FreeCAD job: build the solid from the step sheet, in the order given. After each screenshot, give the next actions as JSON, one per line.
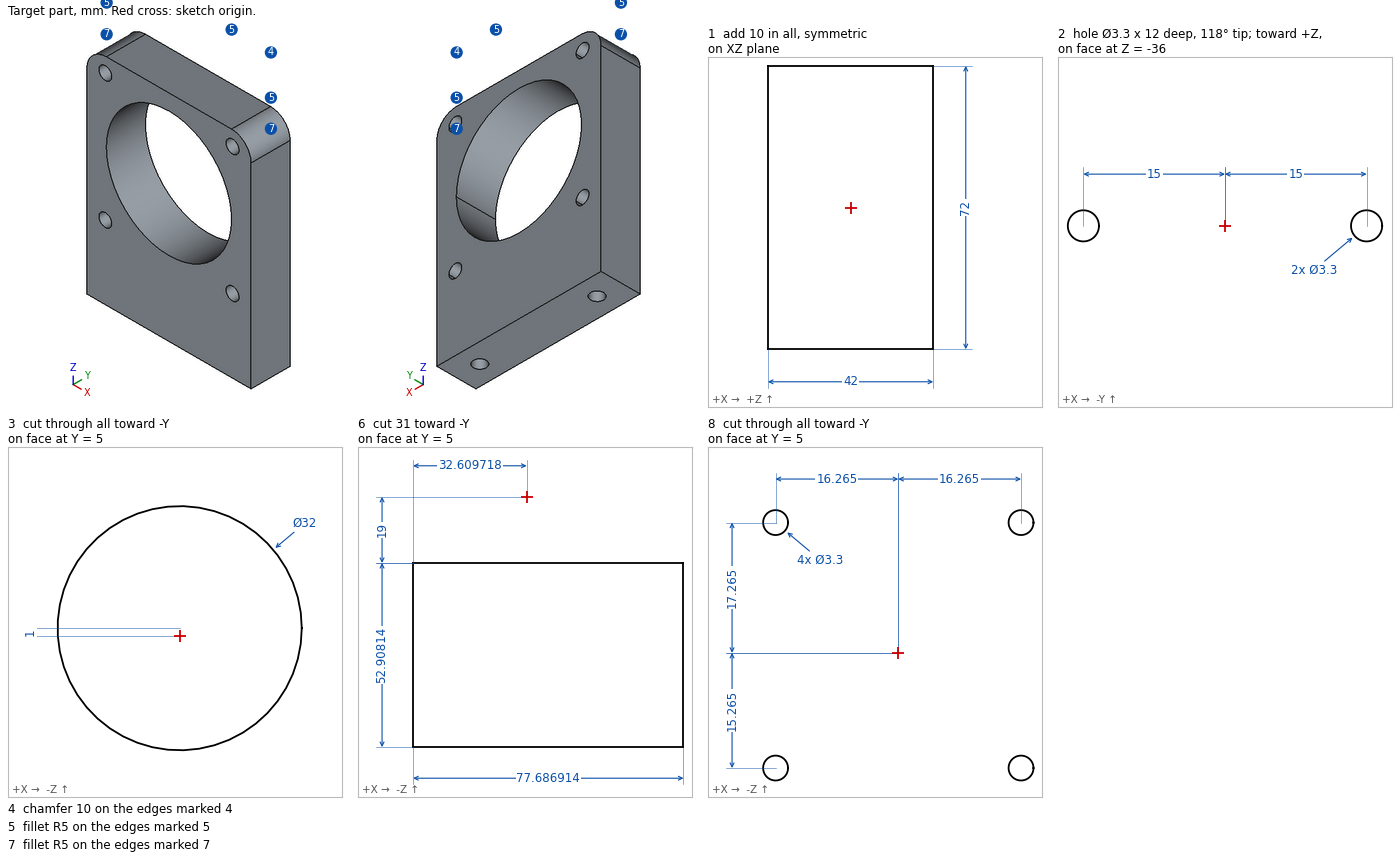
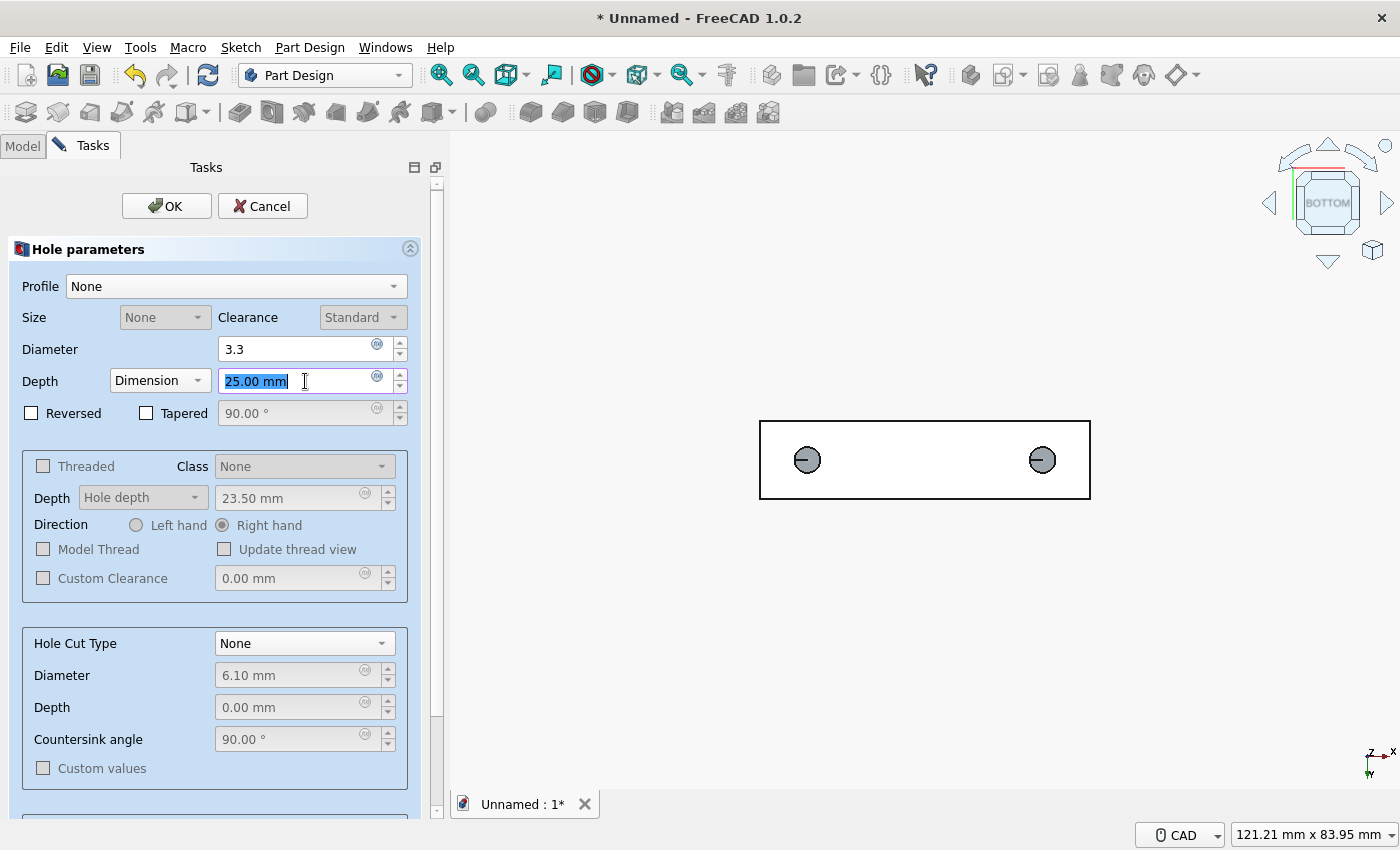
{"action": "type", "text": "12"}
{"action": "key", "text": "Tab"}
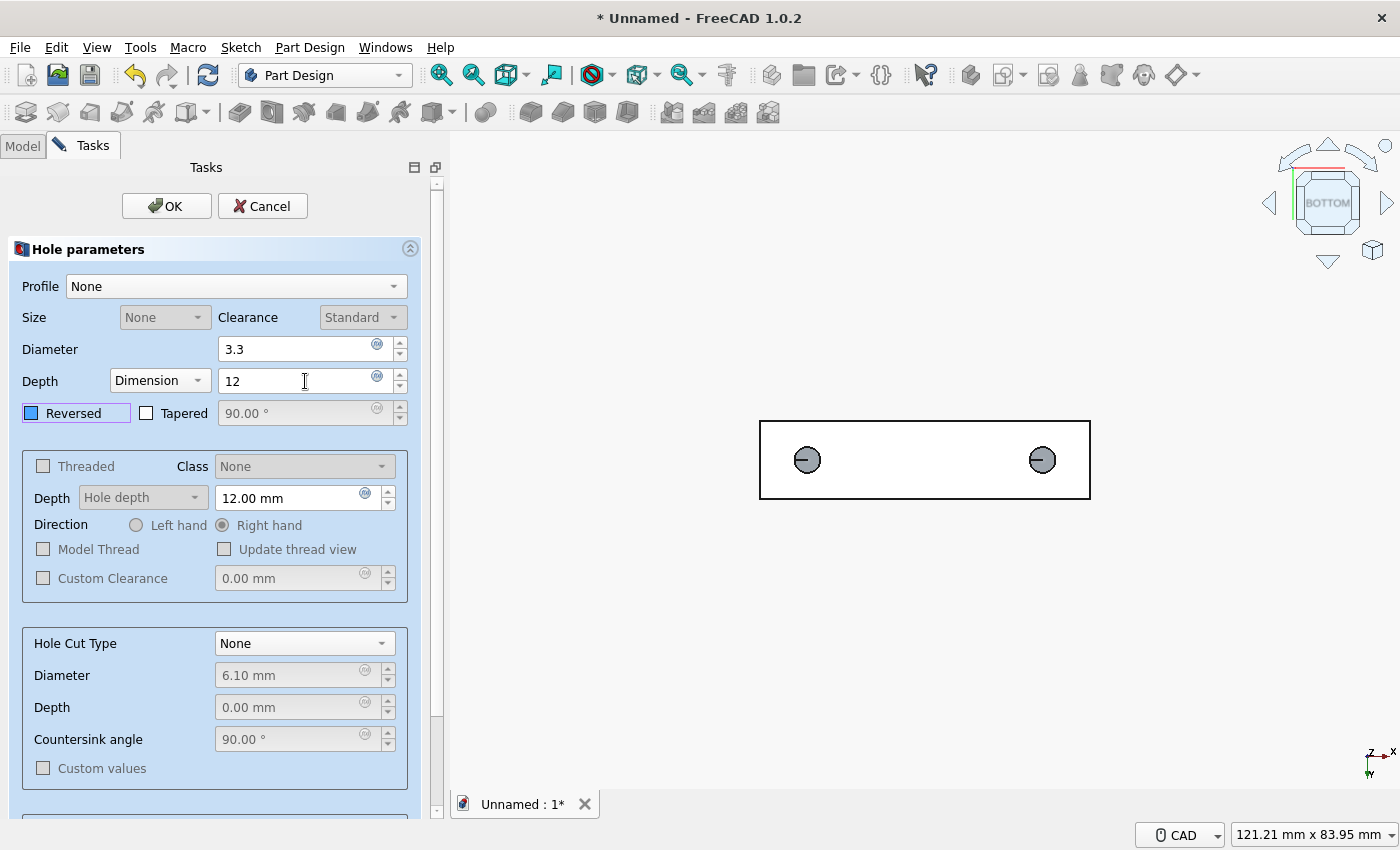
{"action": "left_click", "coordinate": [167, 206]}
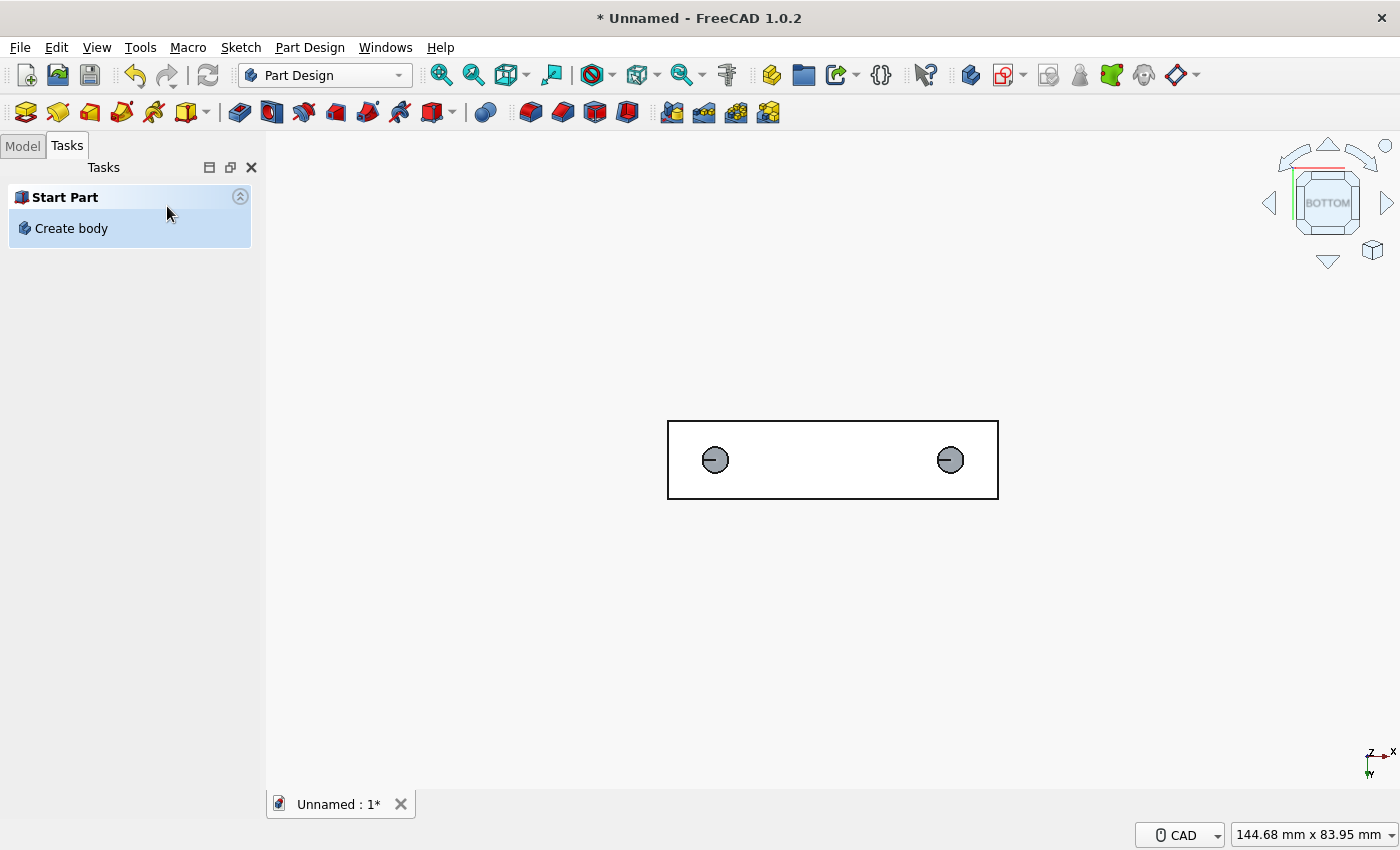
{"action": "left_click", "coordinate": [442, 76]}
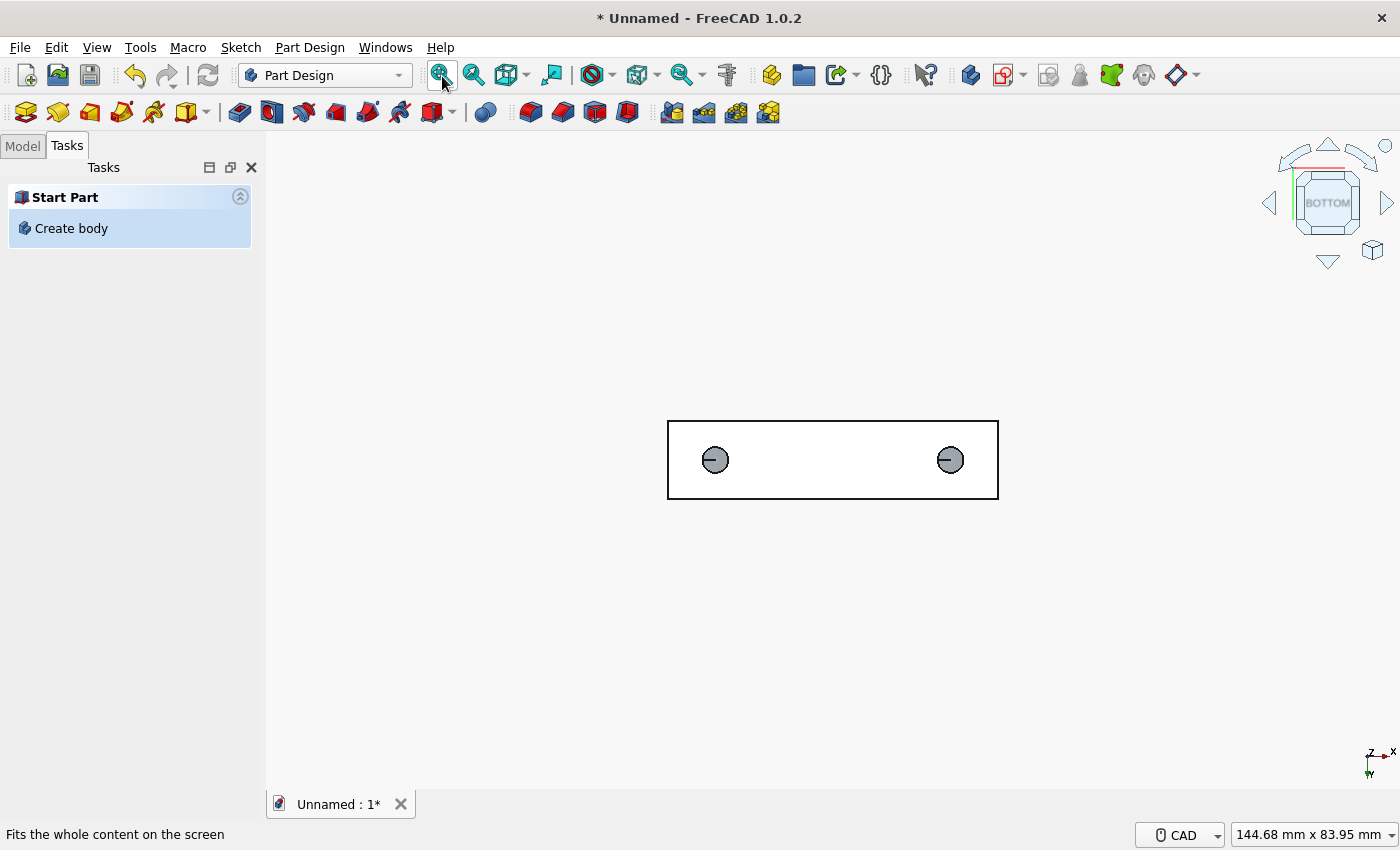
{"action": "key", "text": "4"}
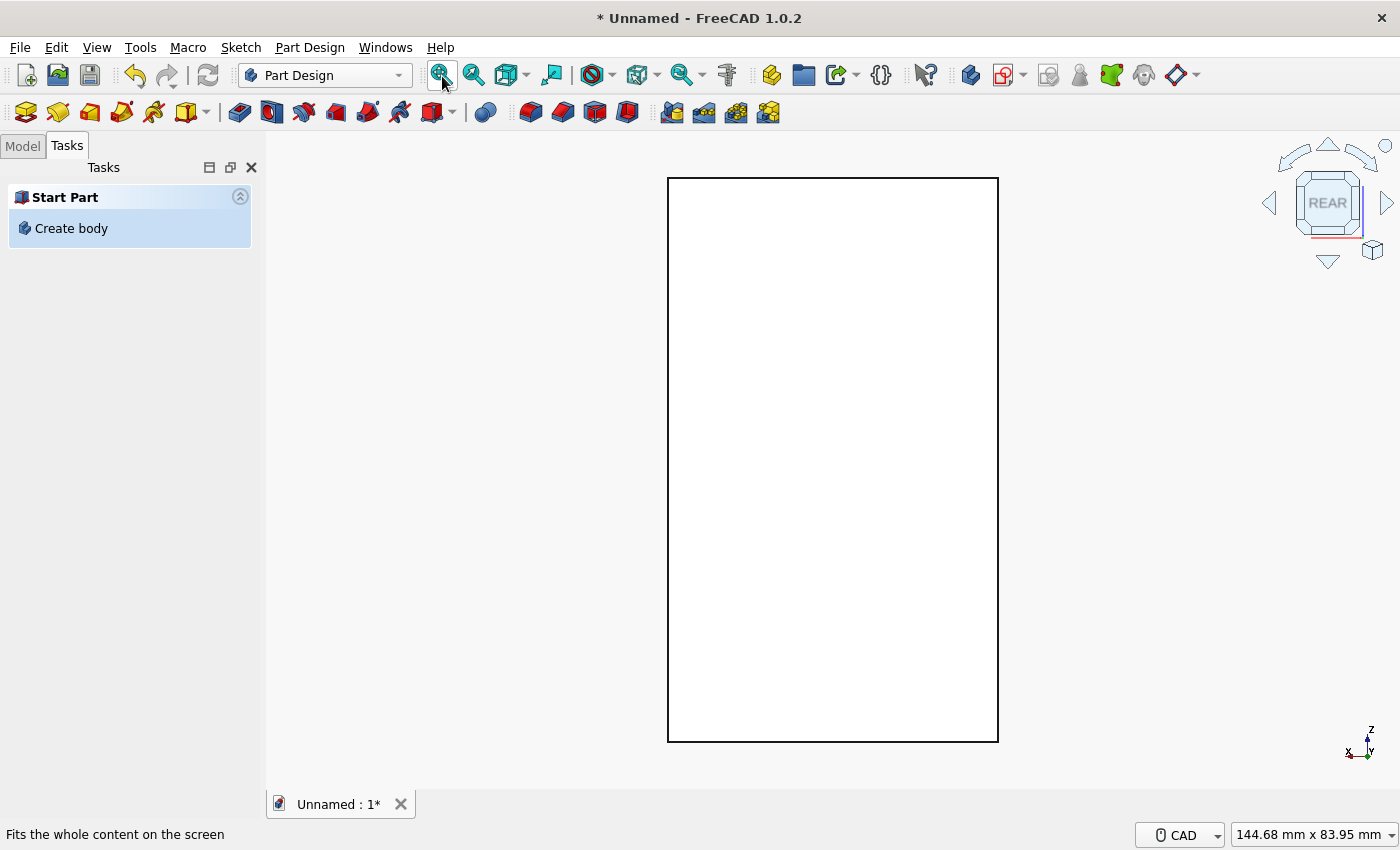
{"action": "left_click", "coordinate": [833, 378]}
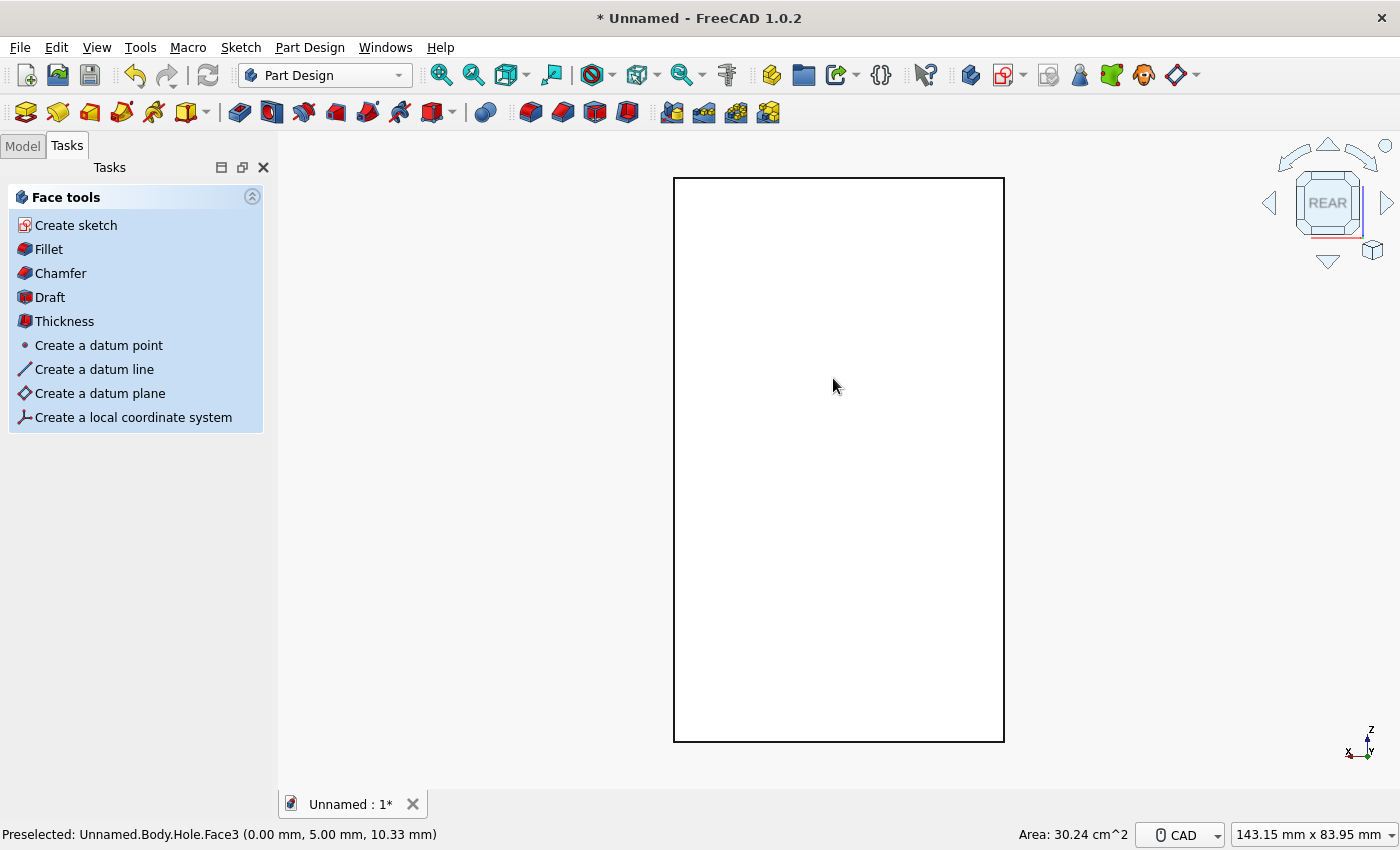
{"action": "left_click", "coordinate": [1004, 76]}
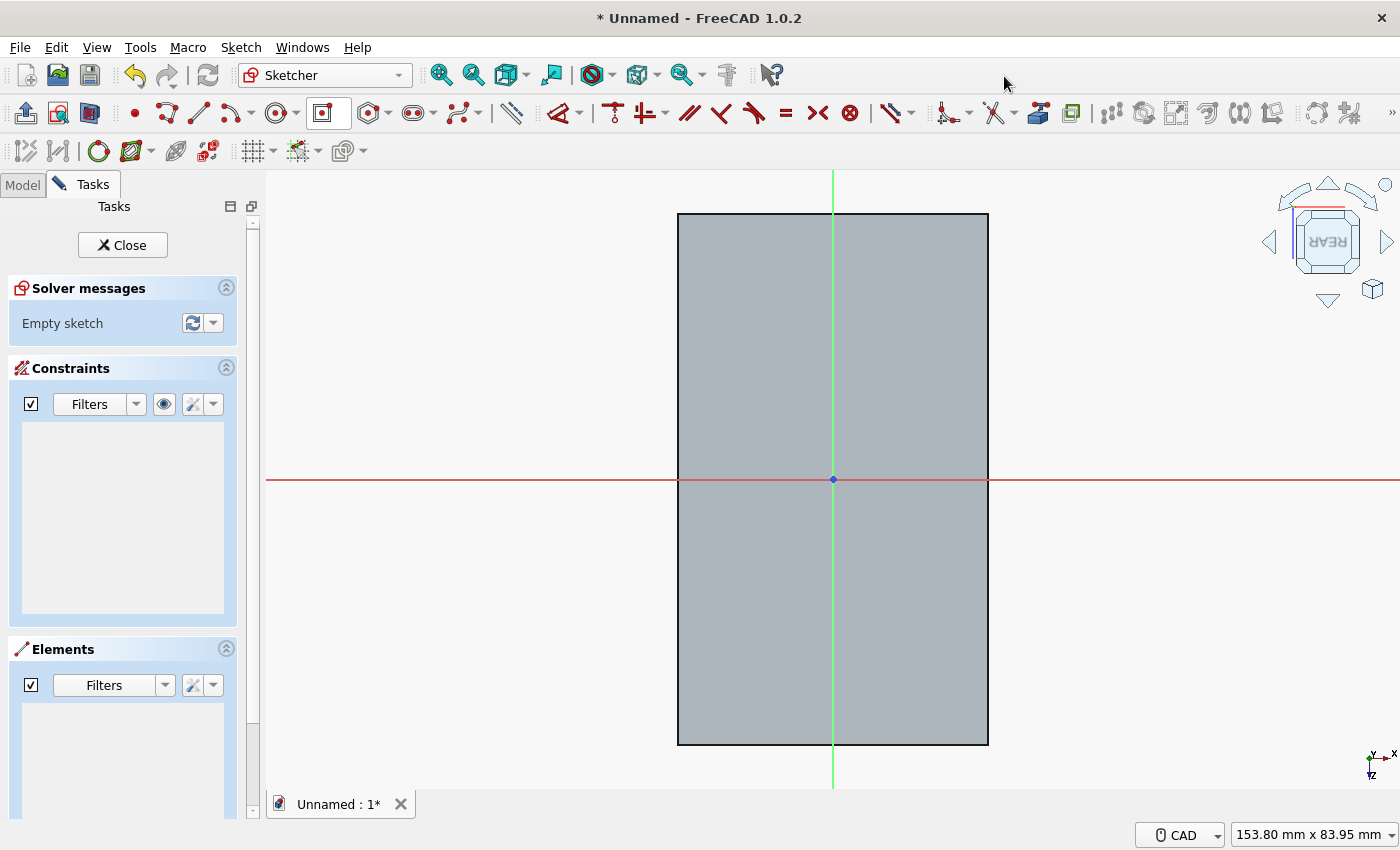
{"action": "scroll", "coordinate": [916, 463], "scroll_direction": "up", "scroll_amount": 3}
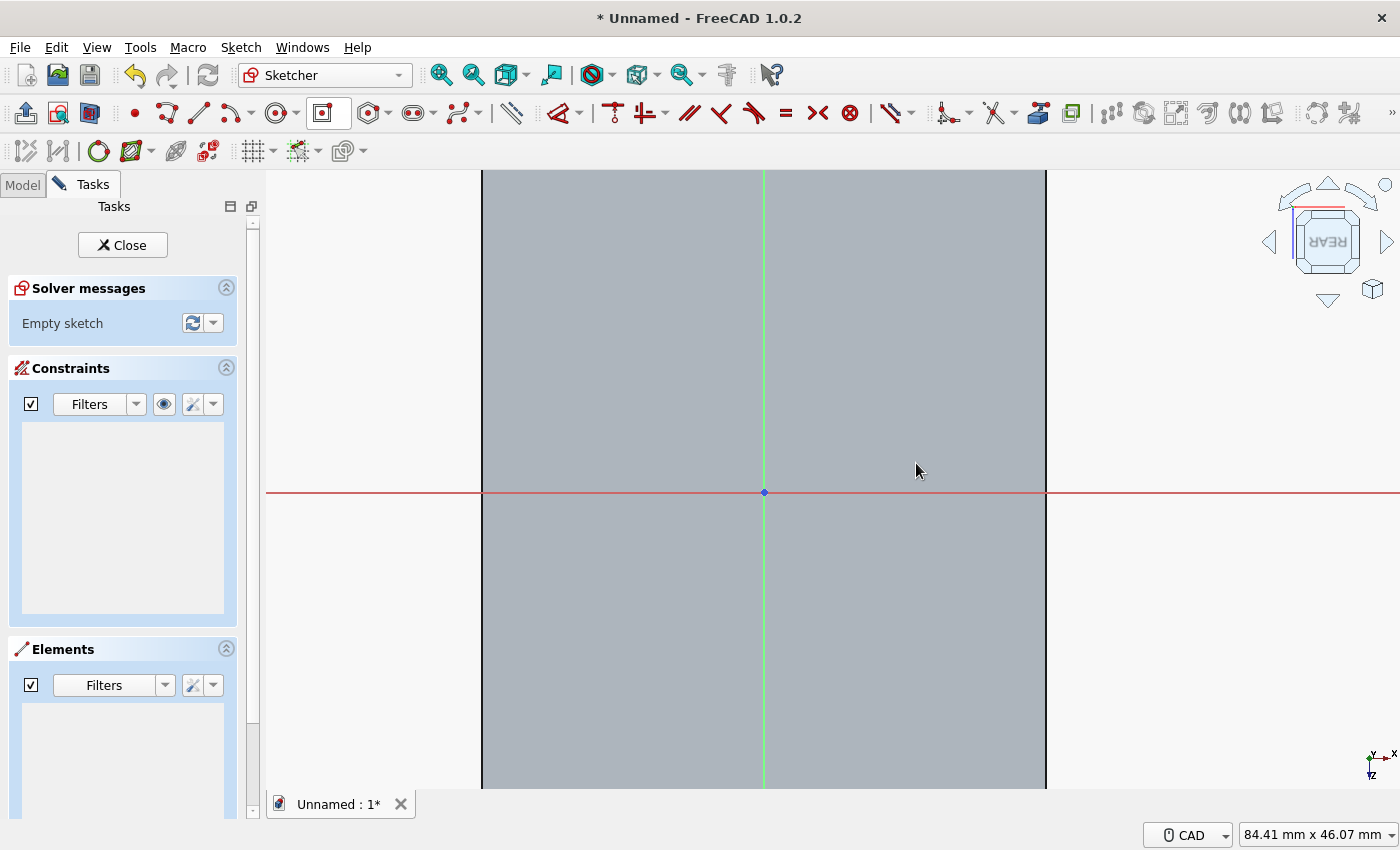
{"action": "left_click", "coordinate": [276, 114]}